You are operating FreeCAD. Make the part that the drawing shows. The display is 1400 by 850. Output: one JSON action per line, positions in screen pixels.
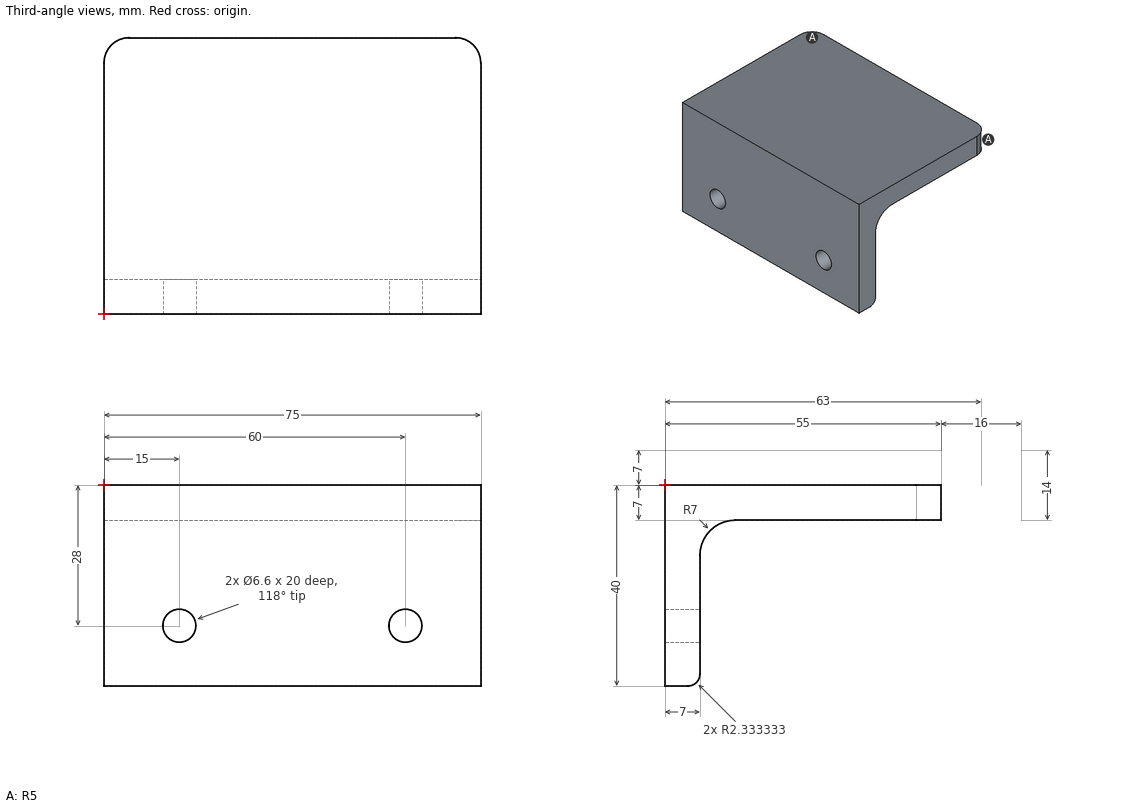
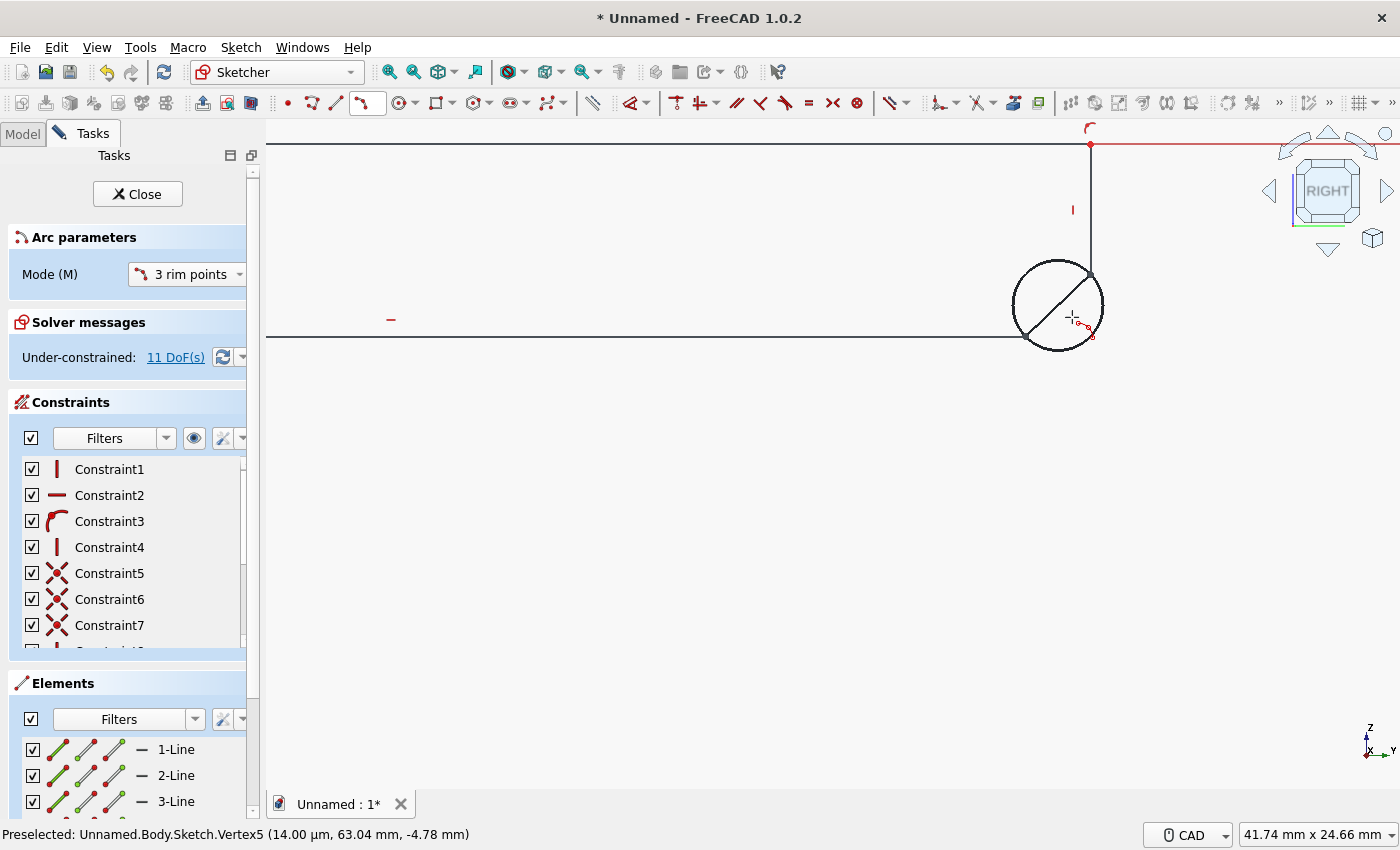
{"action": "left_click", "coordinate": [1071, 316]}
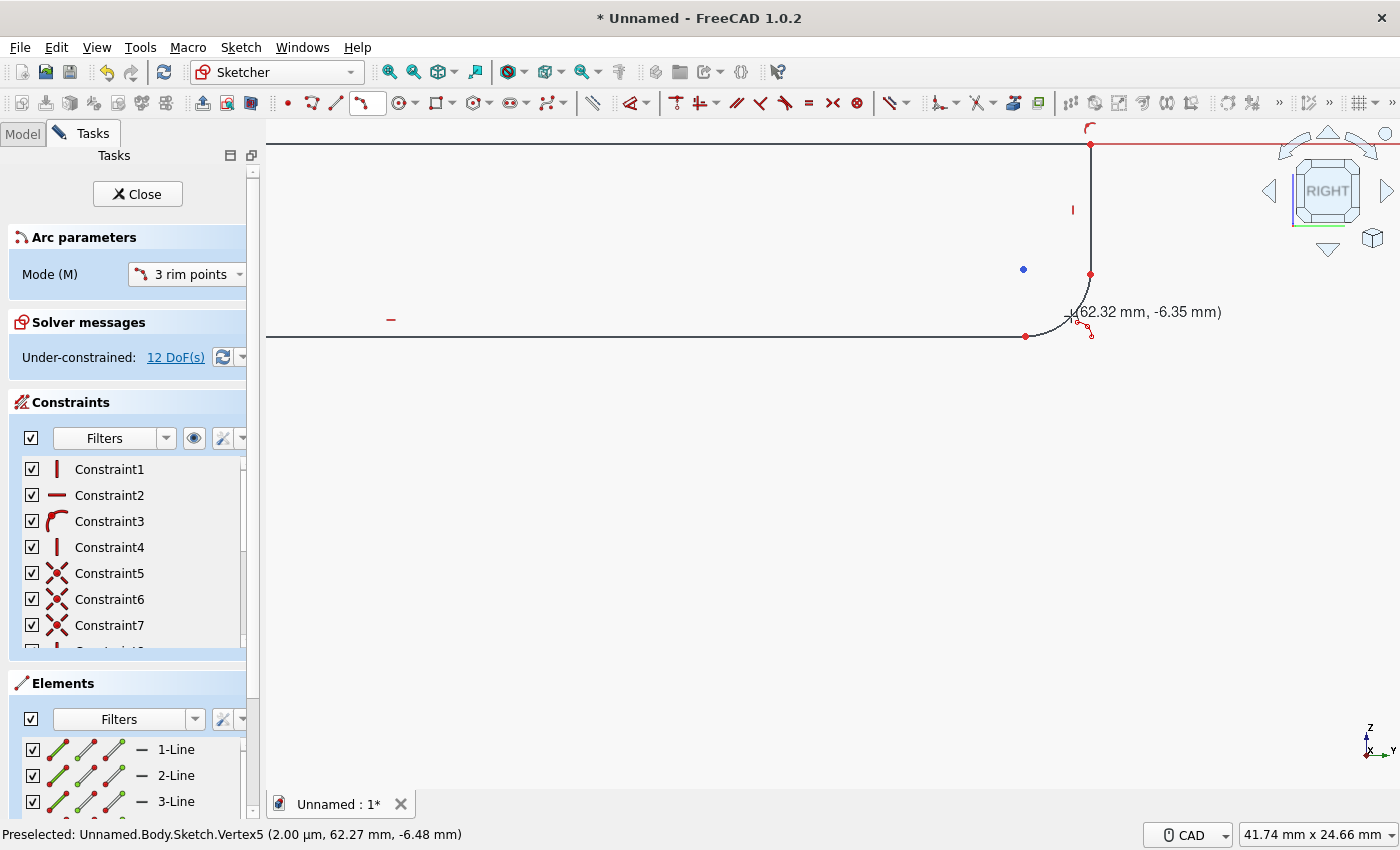
{"action": "scroll", "coordinate": [1073, 318], "scroll_direction": "down", "scroll_amount": 5}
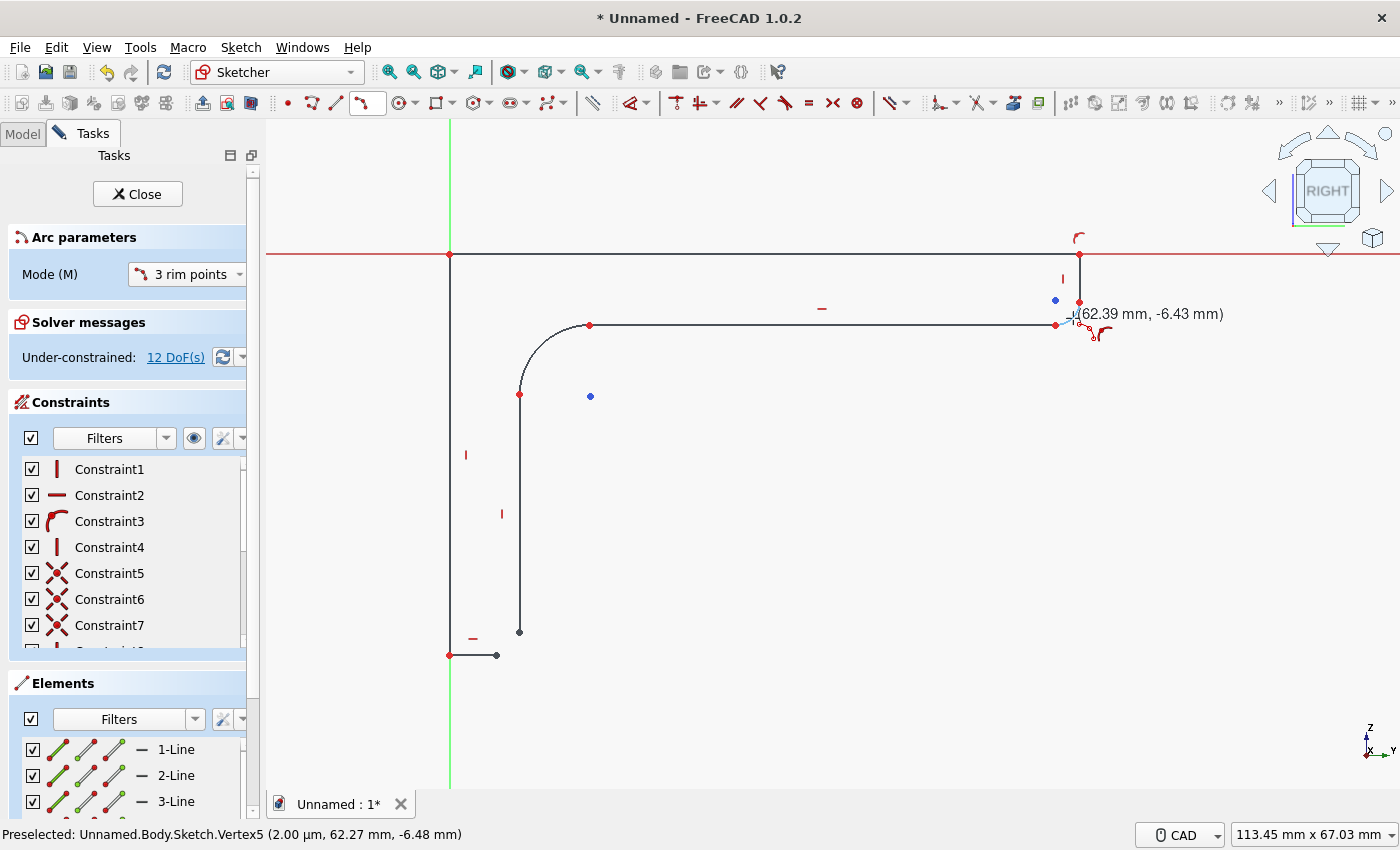
{"action": "left_click", "coordinate": [497, 655]}
{"action": "left_click", "coordinate": [520, 632]}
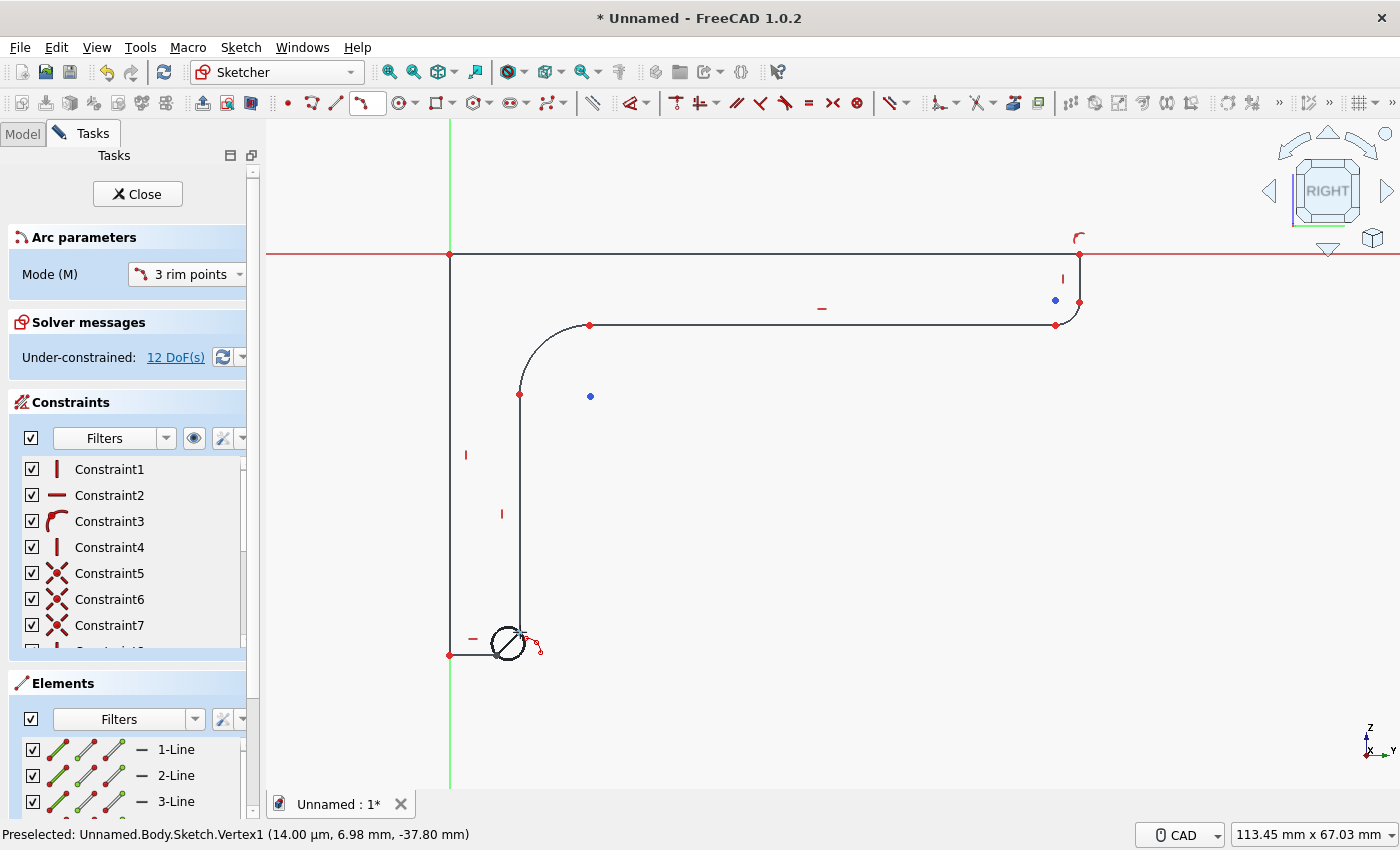
{"action": "scroll", "coordinate": [513, 647], "scroll_direction": "up", "scroll_amount": 5}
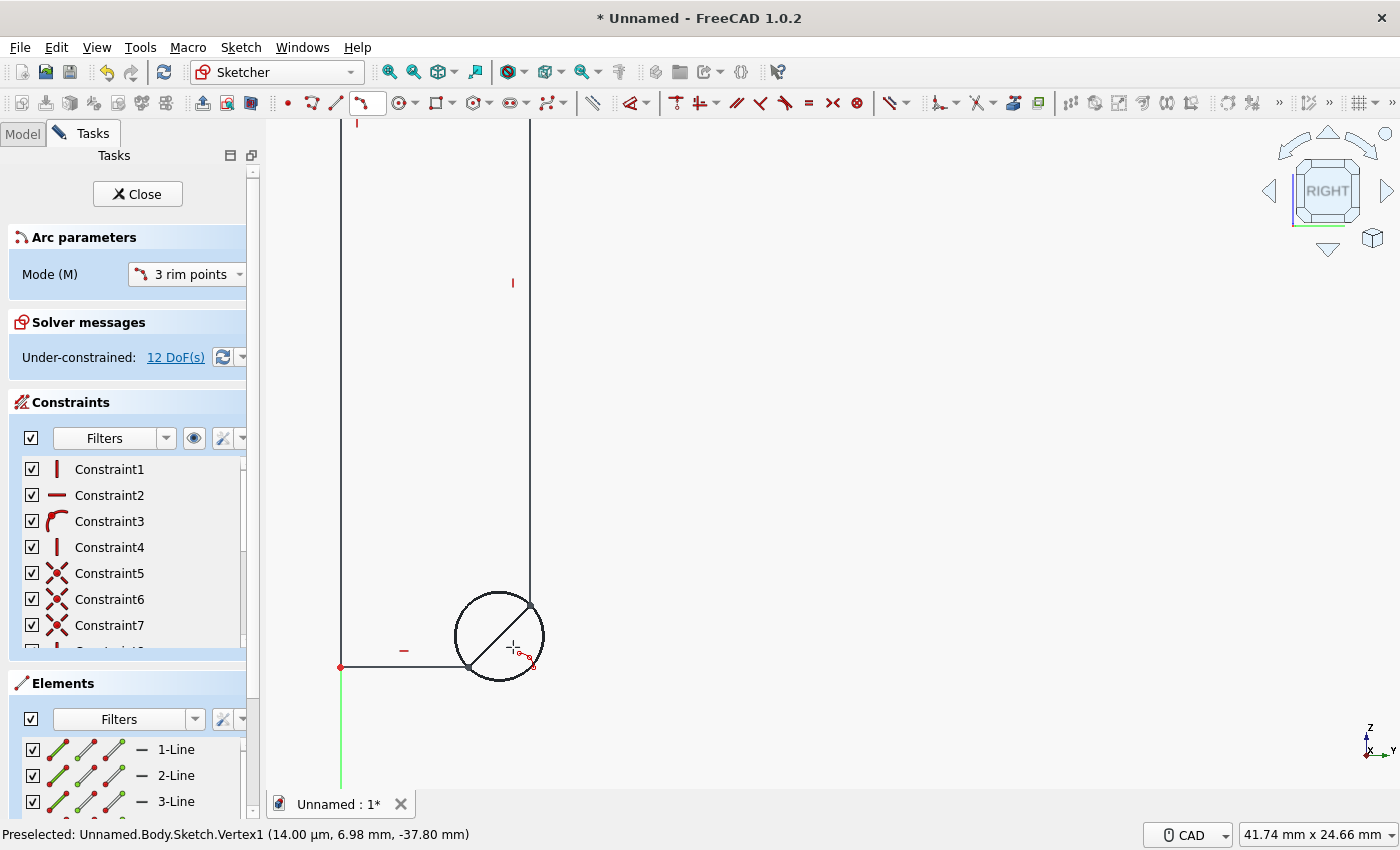
{"action": "left_click", "coordinate": [512, 646]}
{"action": "key", "text": "Escape"}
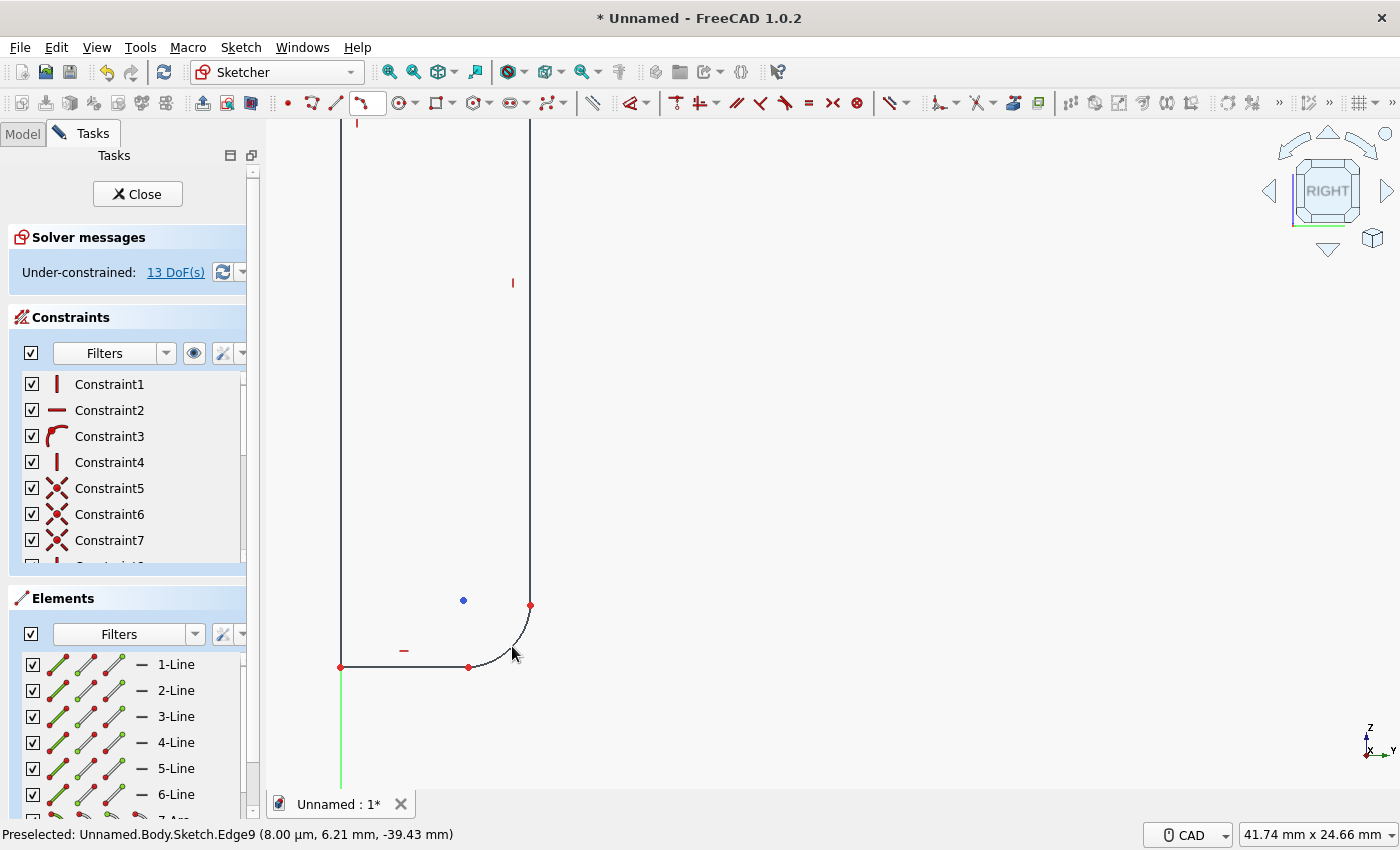
{"action": "left_click", "coordinate": [530, 412]}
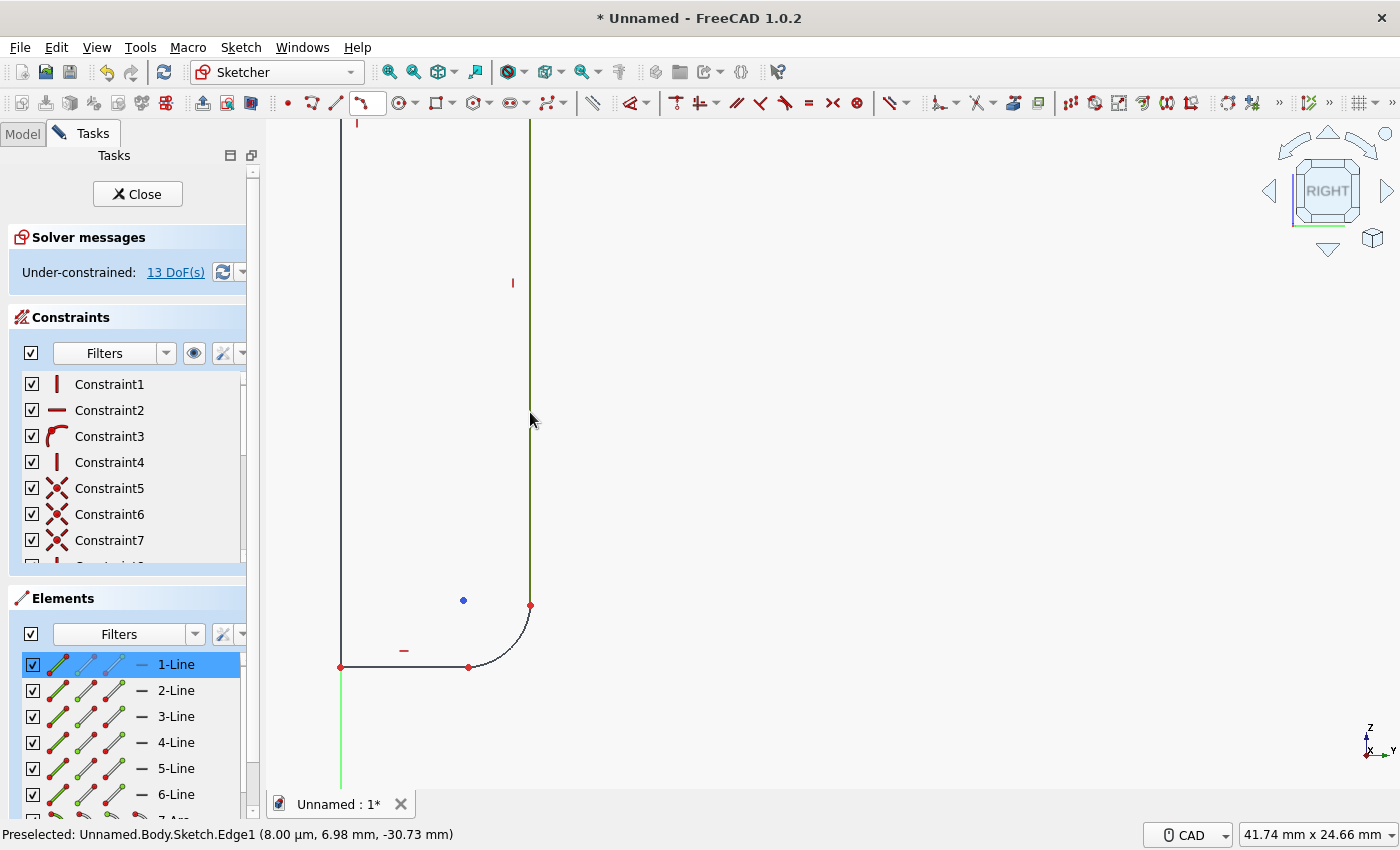
{"action": "scroll", "coordinate": [513, 647], "scroll_direction": "down", "scroll_amount": 5}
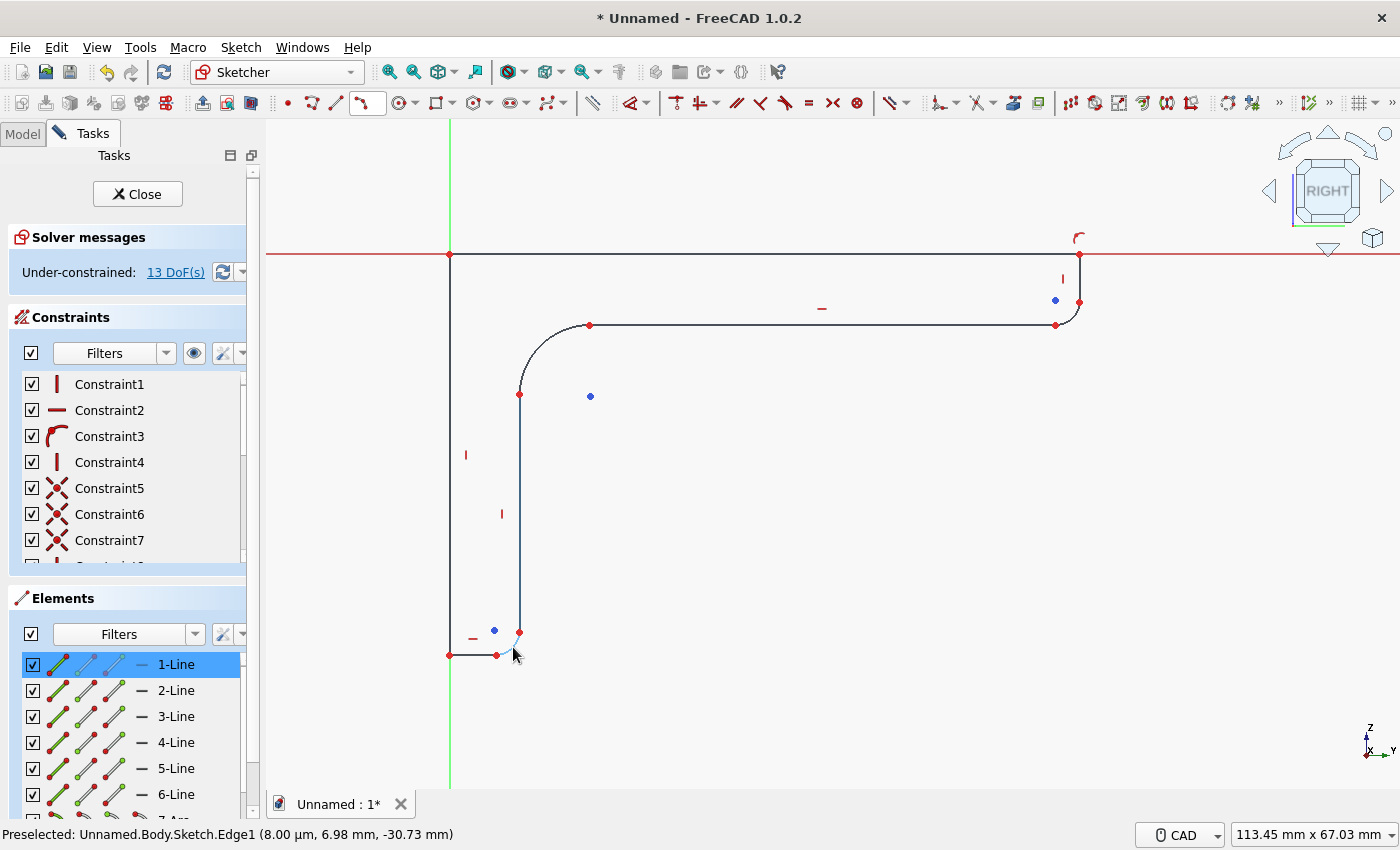
{"action": "left_click", "coordinate": [558, 333]}